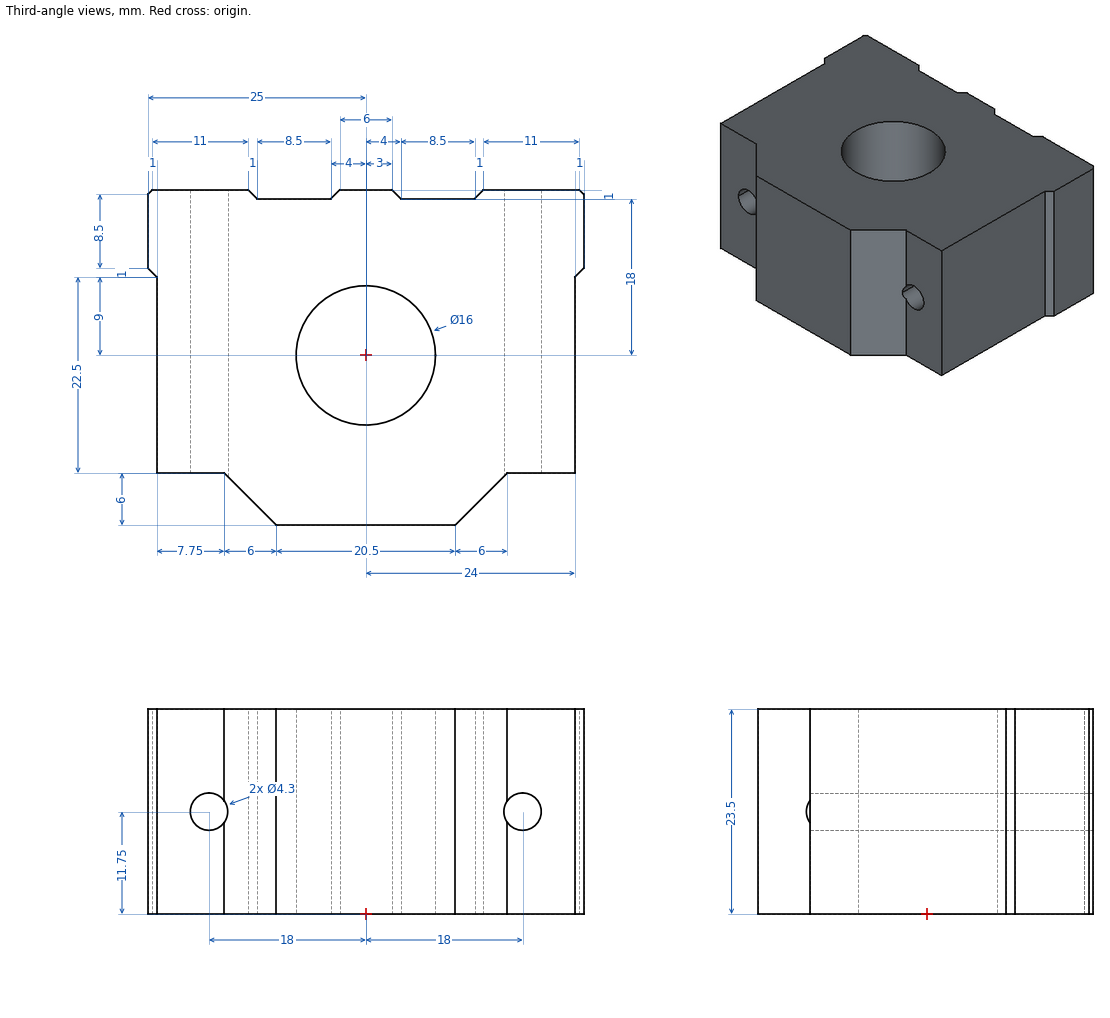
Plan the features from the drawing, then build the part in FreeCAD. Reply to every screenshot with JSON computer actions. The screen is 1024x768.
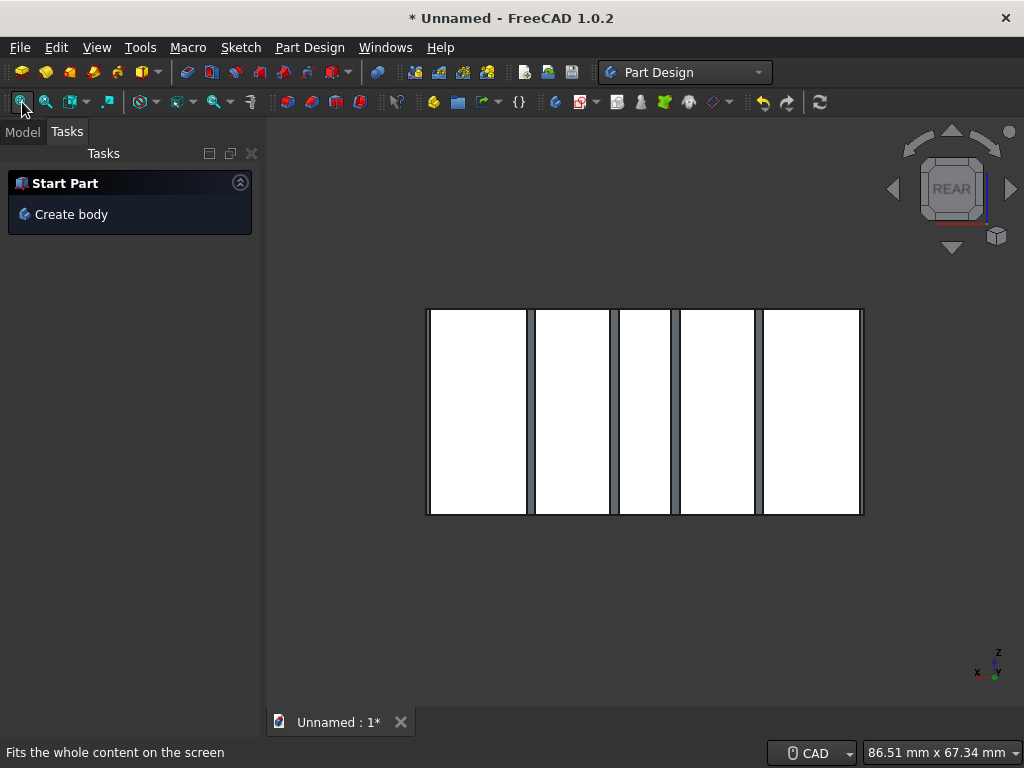
{"action": "left_click", "coordinate": [811, 382]}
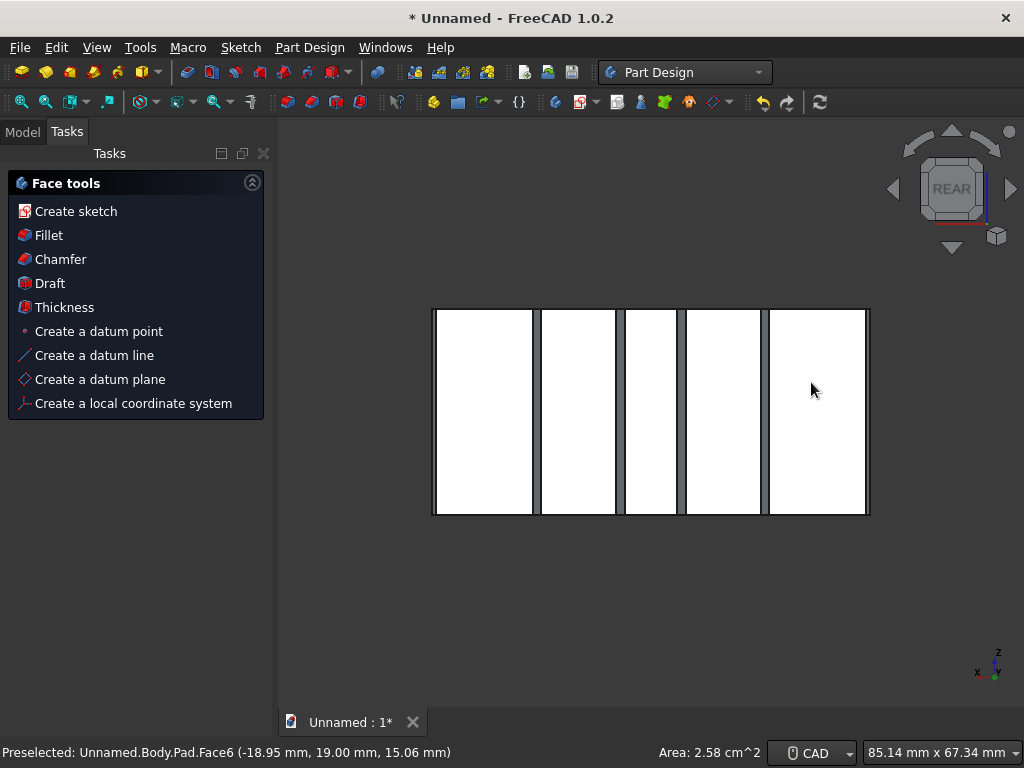
{"action": "left_click", "coordinate": [580, 102]}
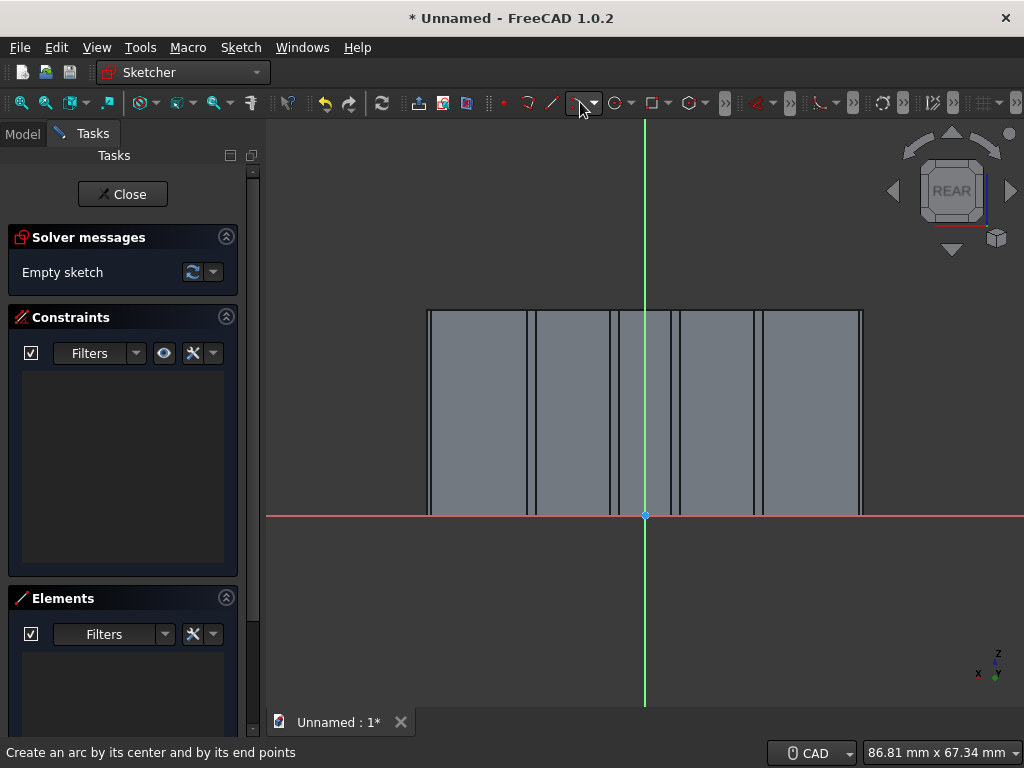
{"action": "left_click", "coordinate": [616, 104]}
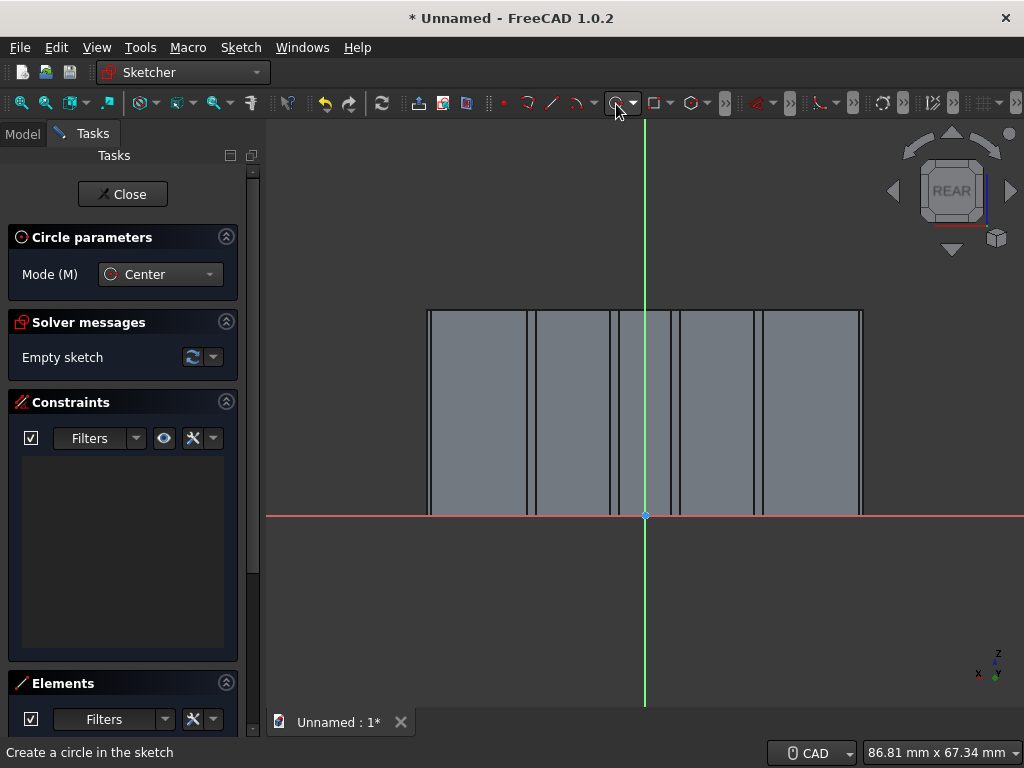
{"action": "left_click", "coordinate": [802, 413]}
{"action": "mouse_move", "coordinate": [815, 400]}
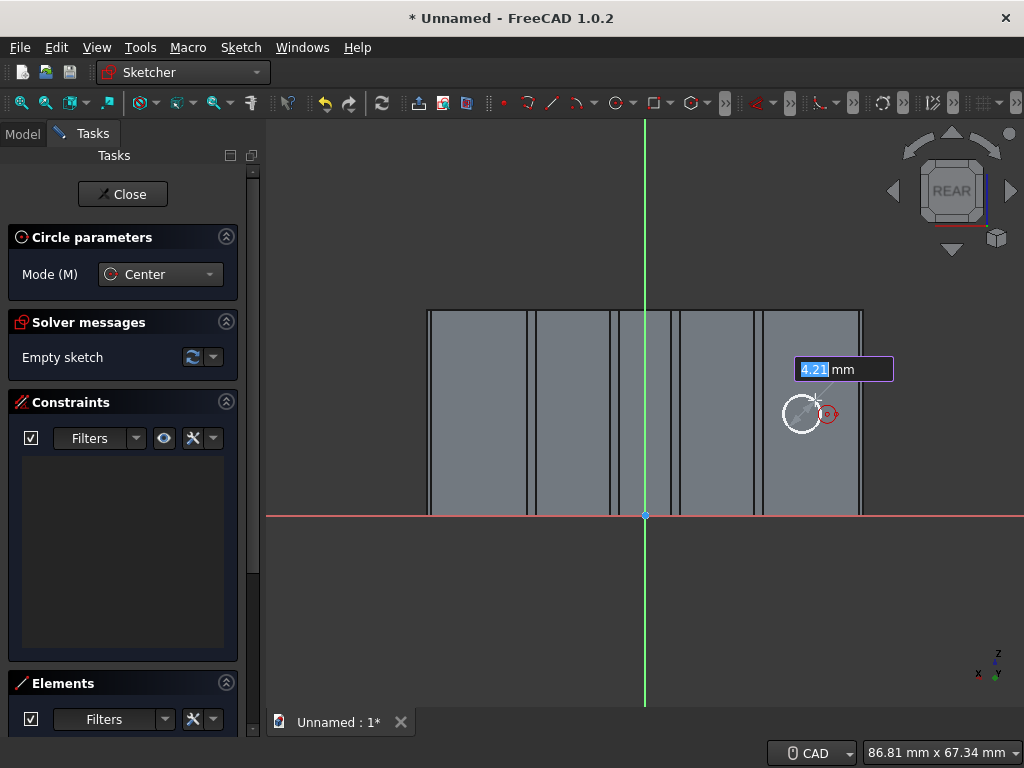
{"action": "type", "text": "4.3"}
{"action": "key", "text": "Return"}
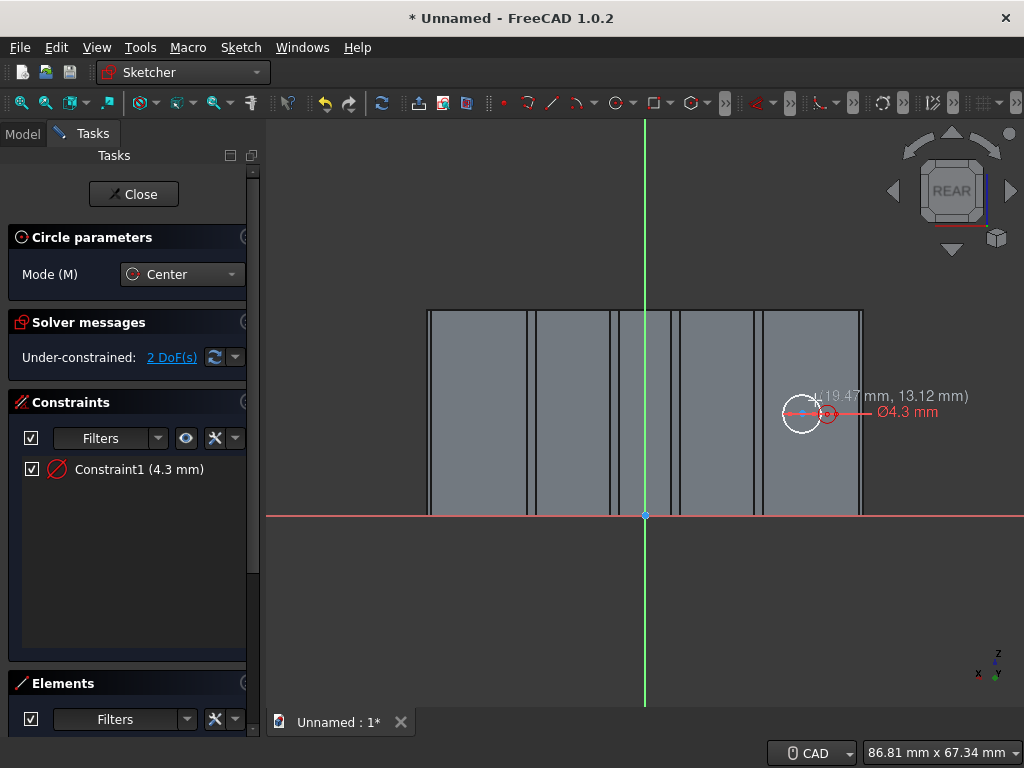
{"action": "left_click", "coordinate": [488, 413]}
{"action": "mouse_move", "coordinate": [501, 400]}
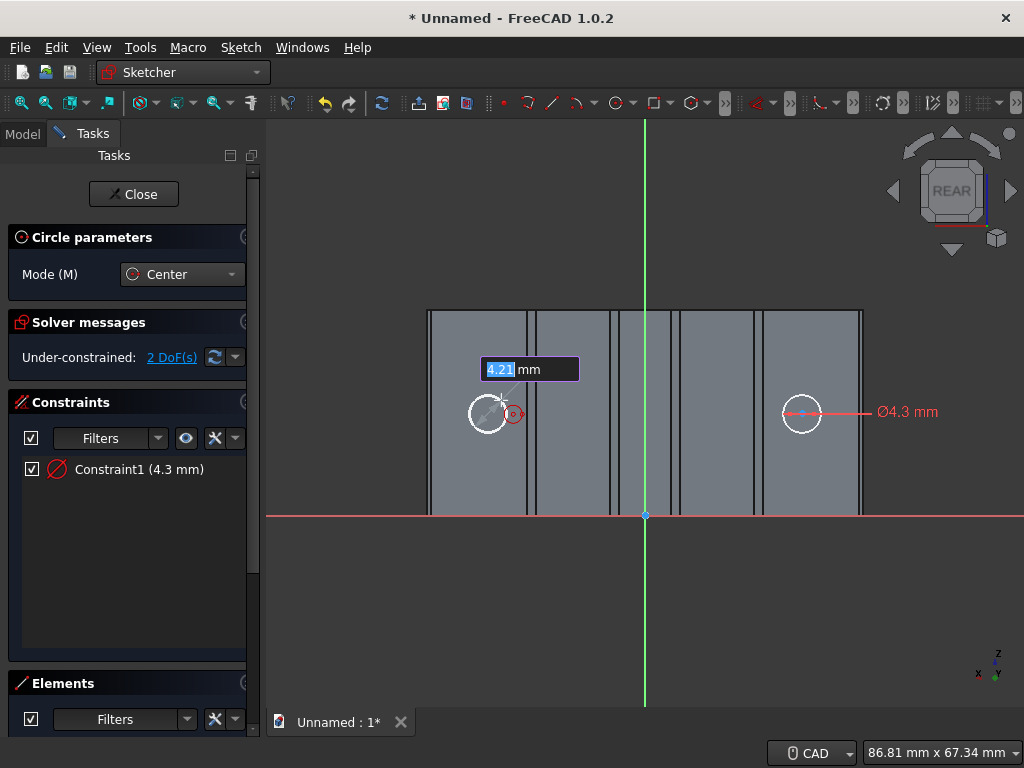
{"action": "type", "text": "4.3"}
{"action": "key", "text": "Return"}
{"action": "key", "text": "Escape"}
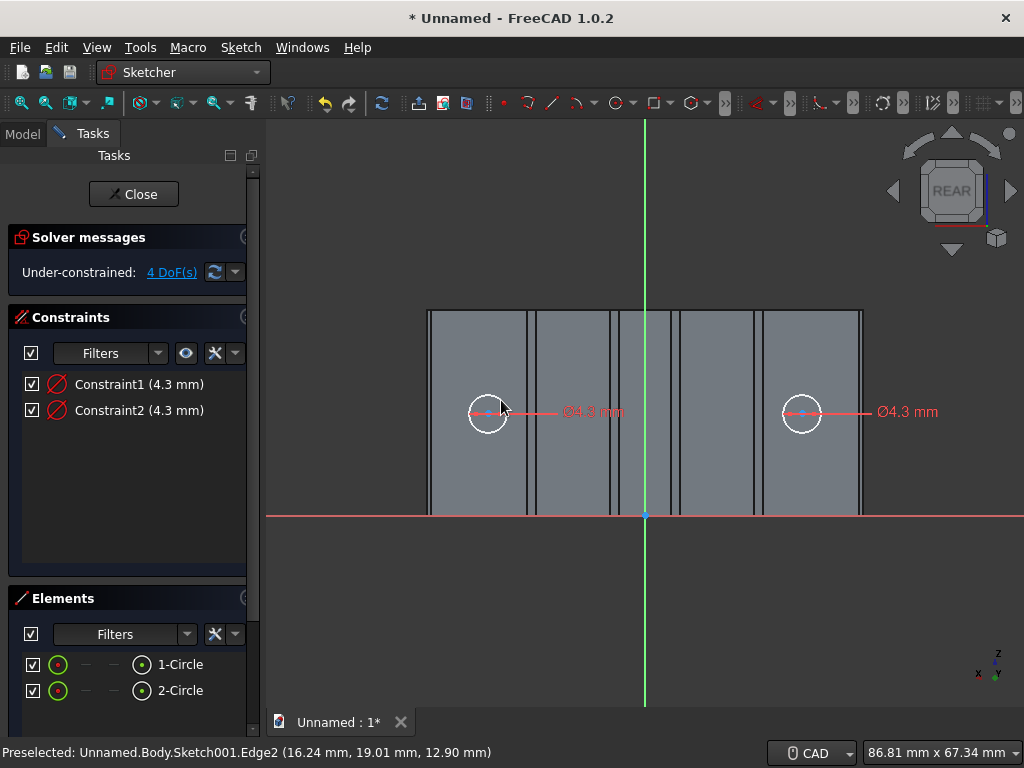
{"action": "left_click", "coordinate": [802, 414]}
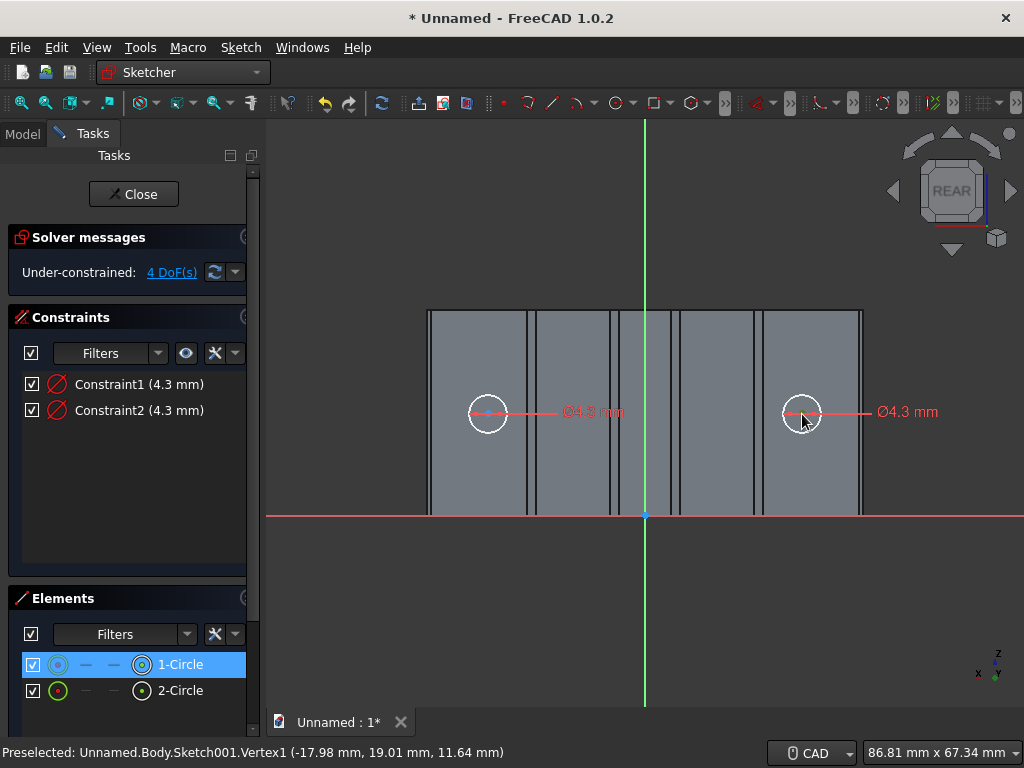
{"action": "left_click", "coordinate": [488, 414]}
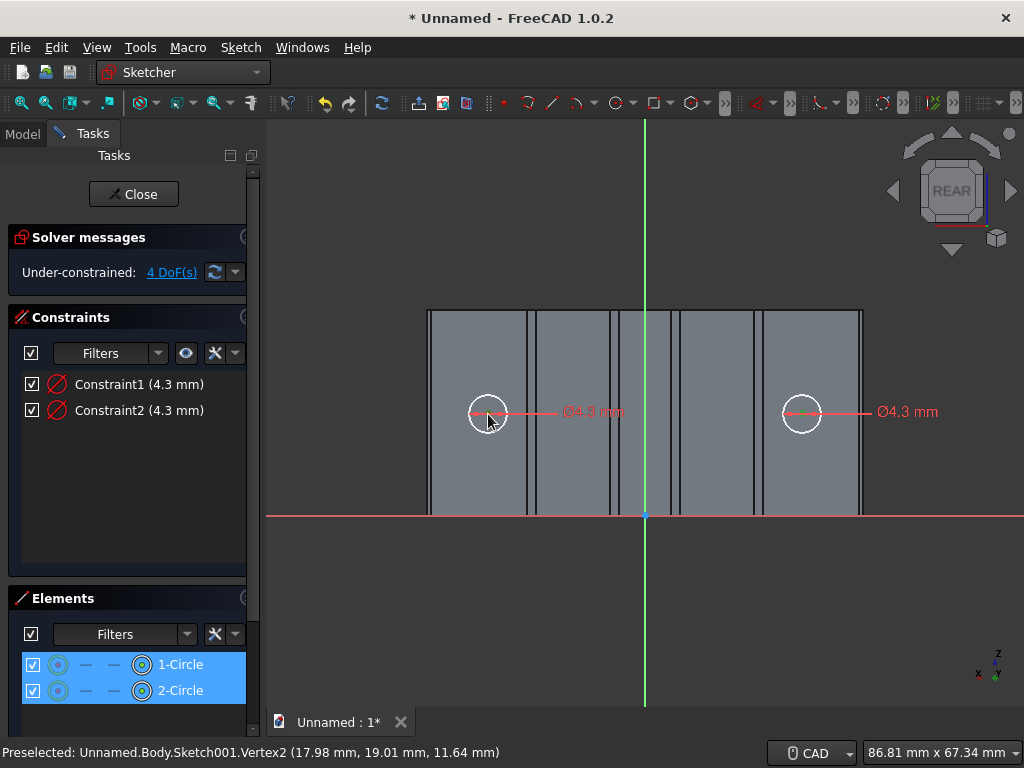
{"action": "key", "text": "h"}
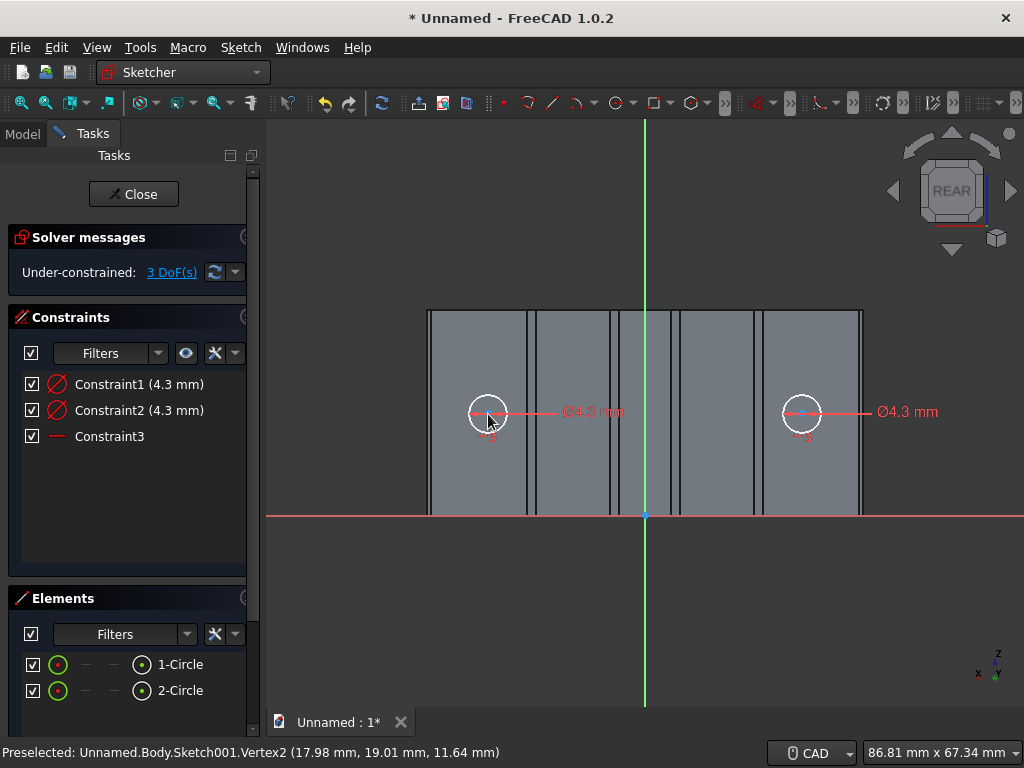
{"action": "left_click", "coordinate": [756, 104]}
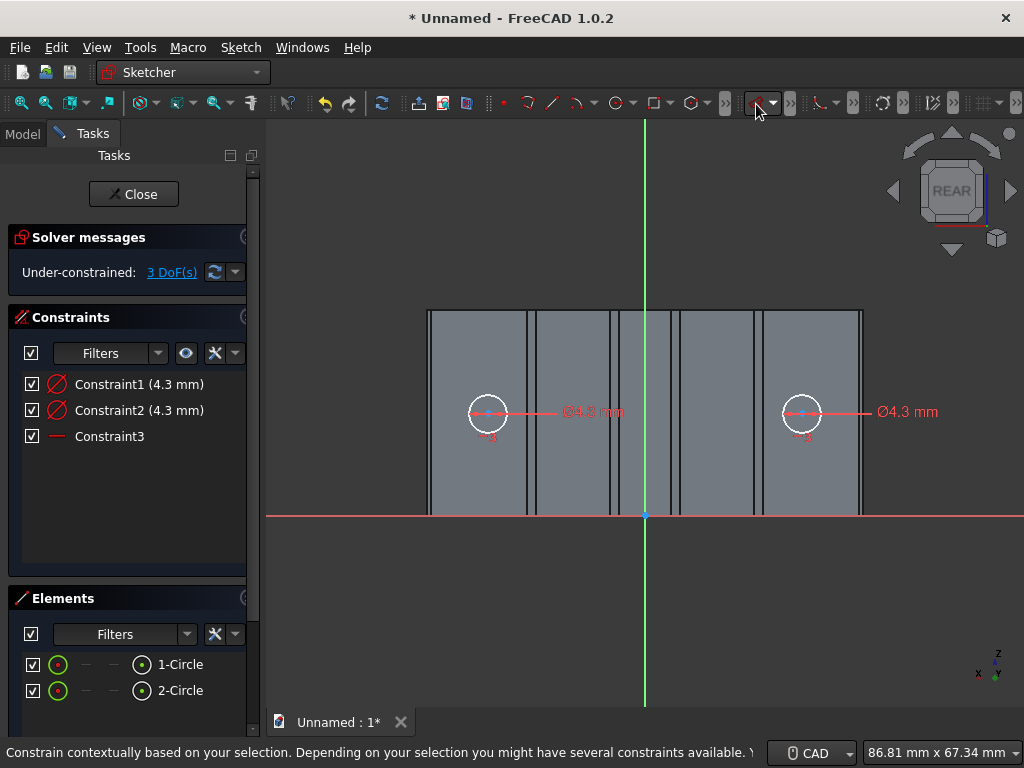
{"action": "left_click", "coordinate": [802, 414]}
{"action": "left_click", "coordinate": [723, 550]}